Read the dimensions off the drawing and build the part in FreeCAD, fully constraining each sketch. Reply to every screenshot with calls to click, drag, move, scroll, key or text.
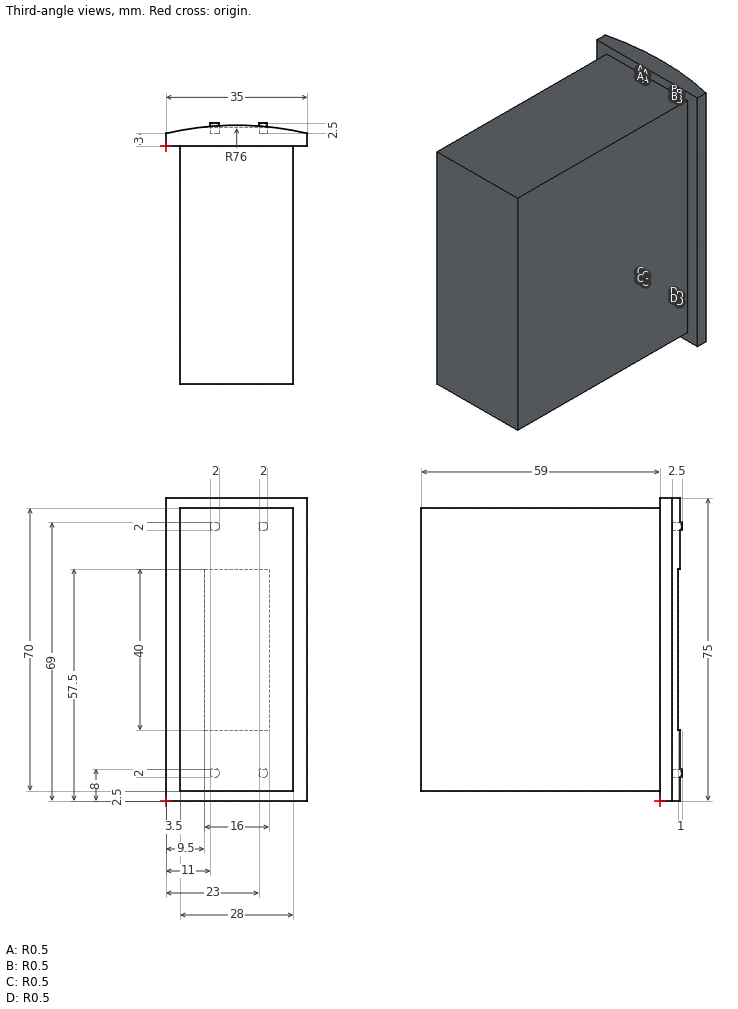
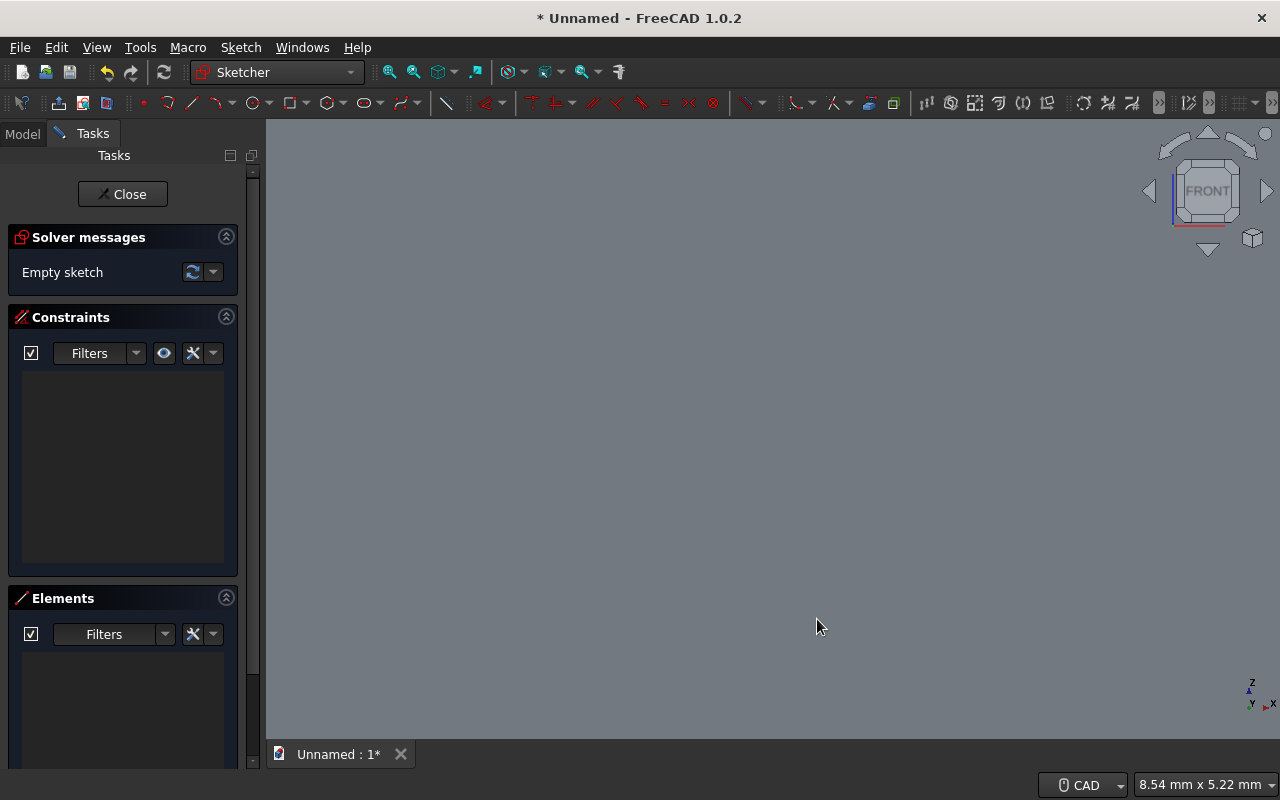
scroll(682, 380, up, 3)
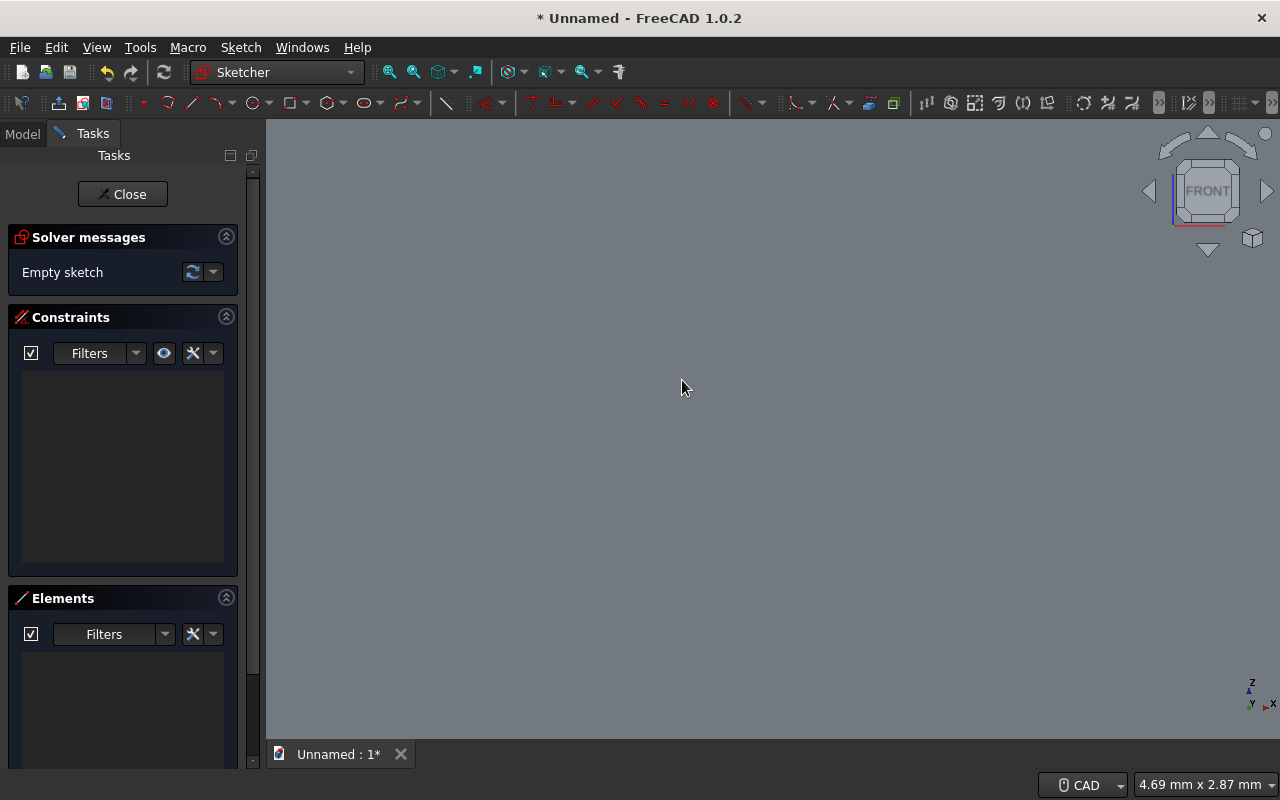
click(290, 104)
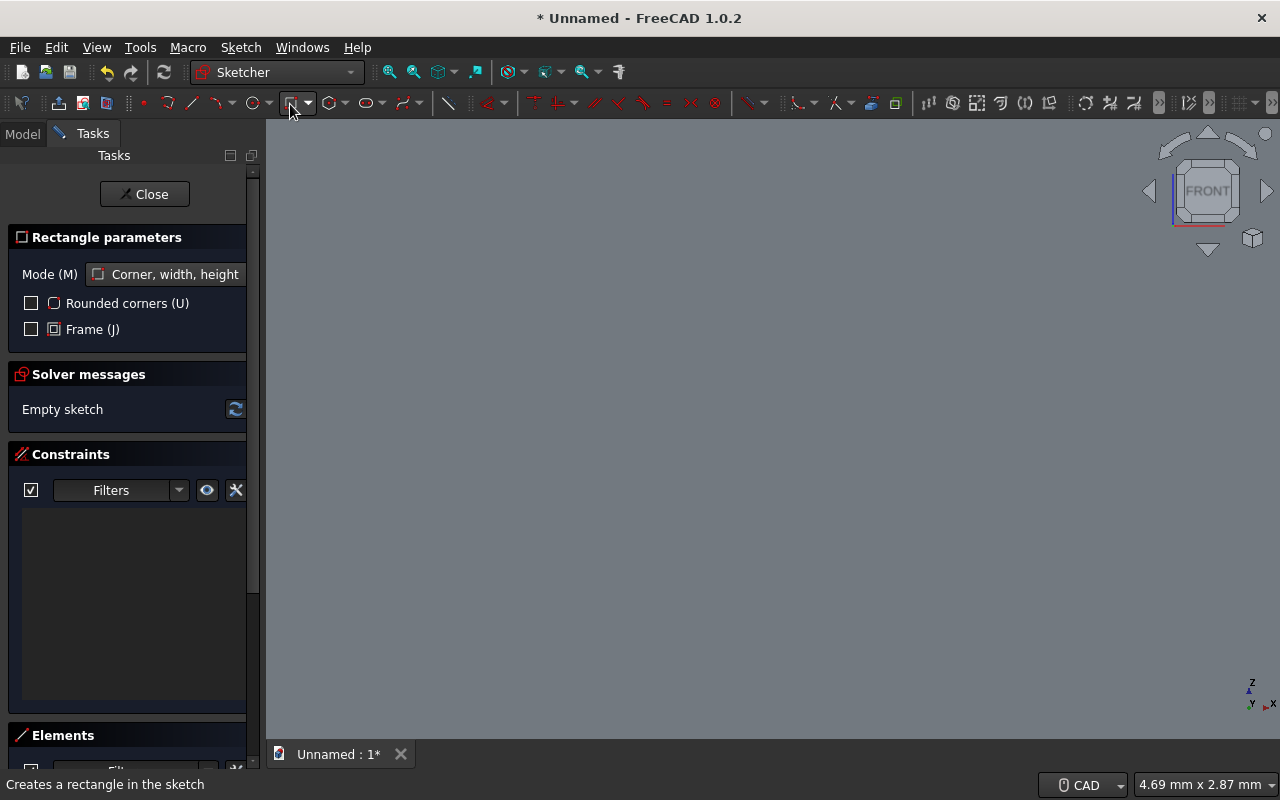
click(488, 213)
click(920, 645)
key(Escape)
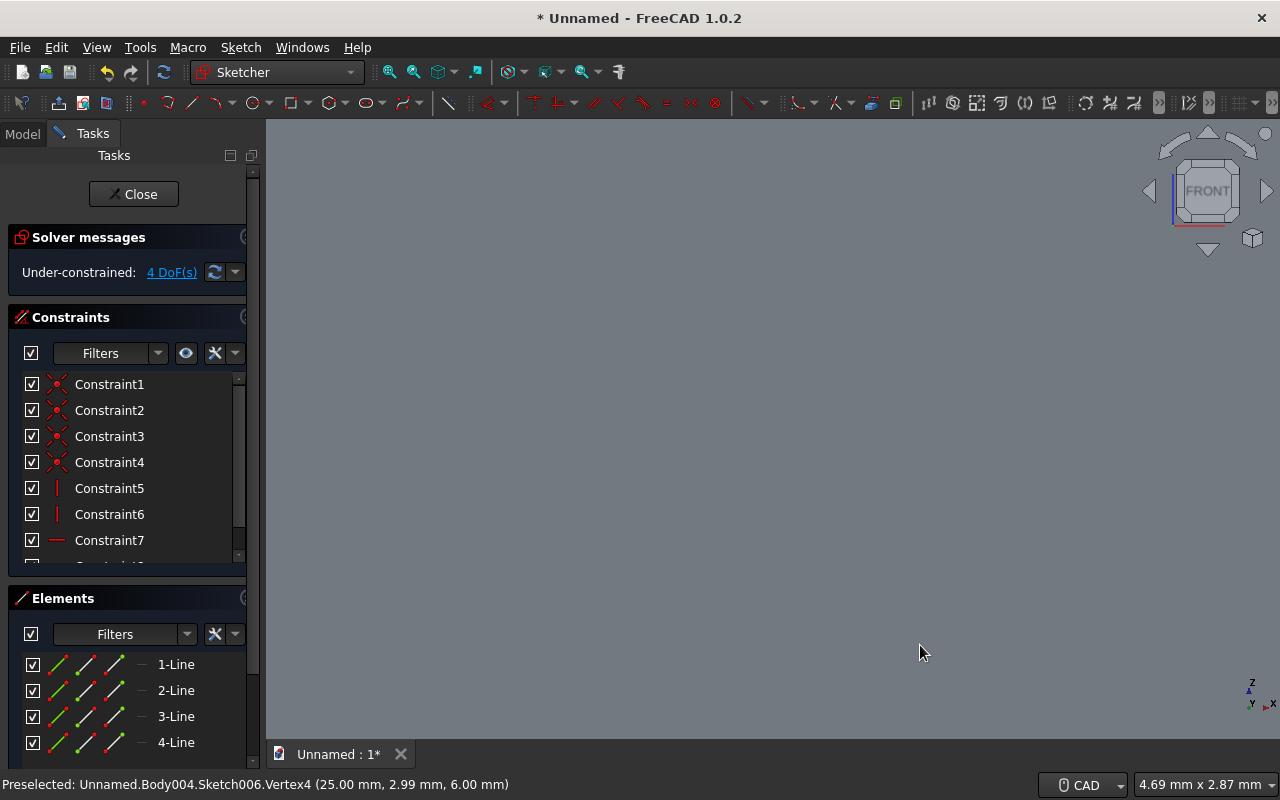
key(d)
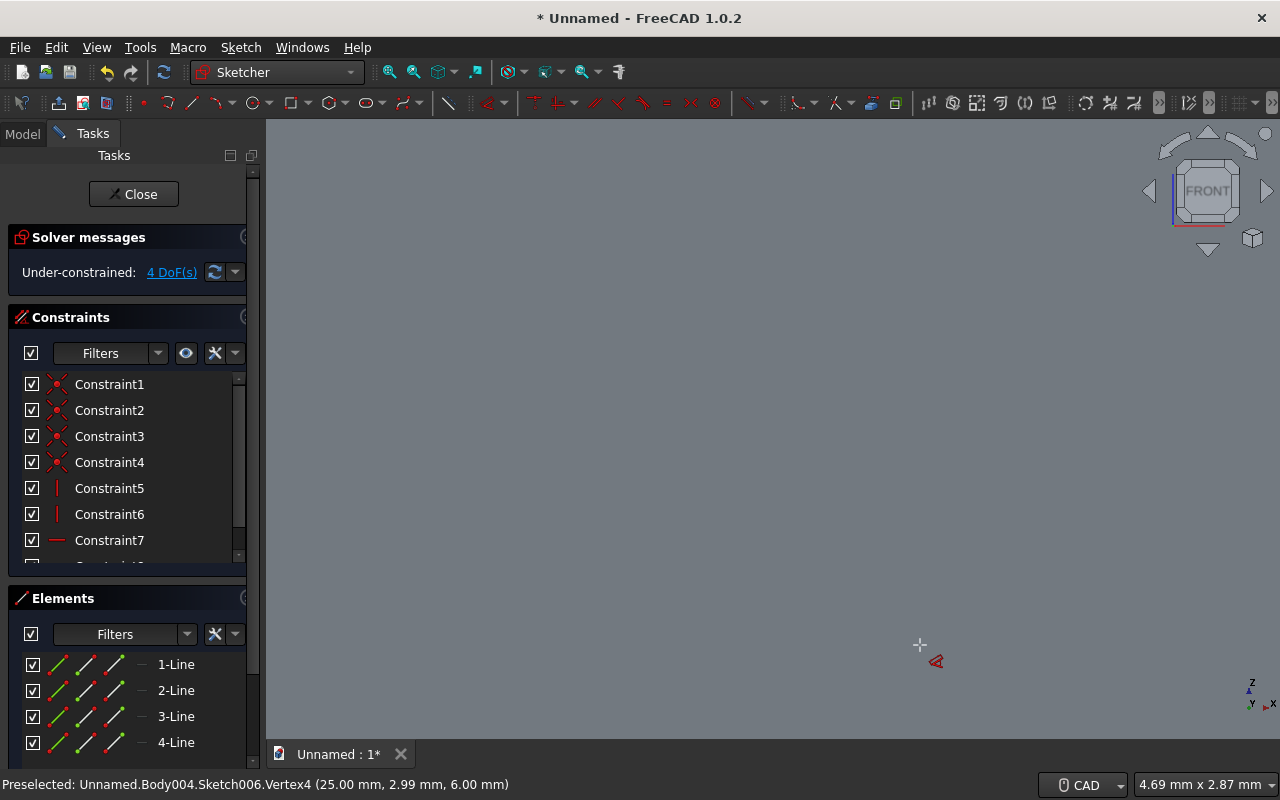
click(488, 344)
click(454, 430)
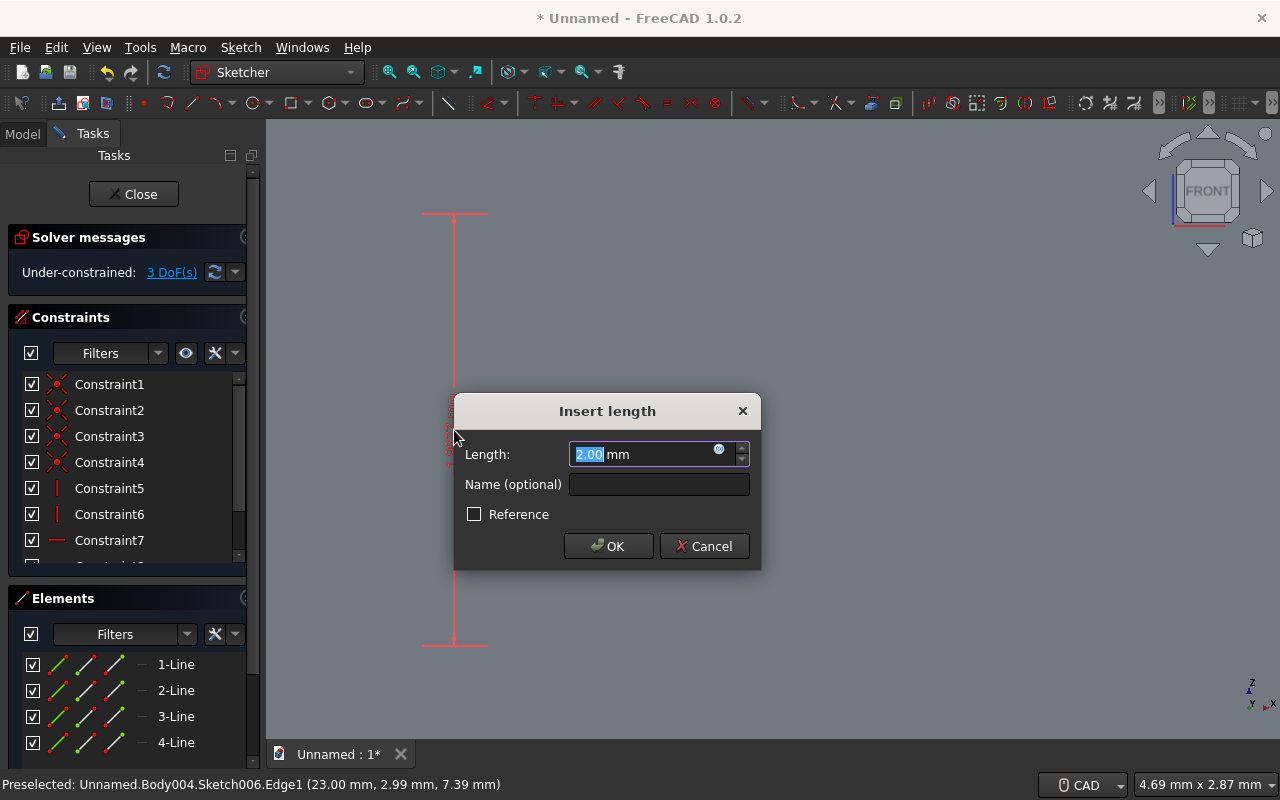
text(2)
key(Return)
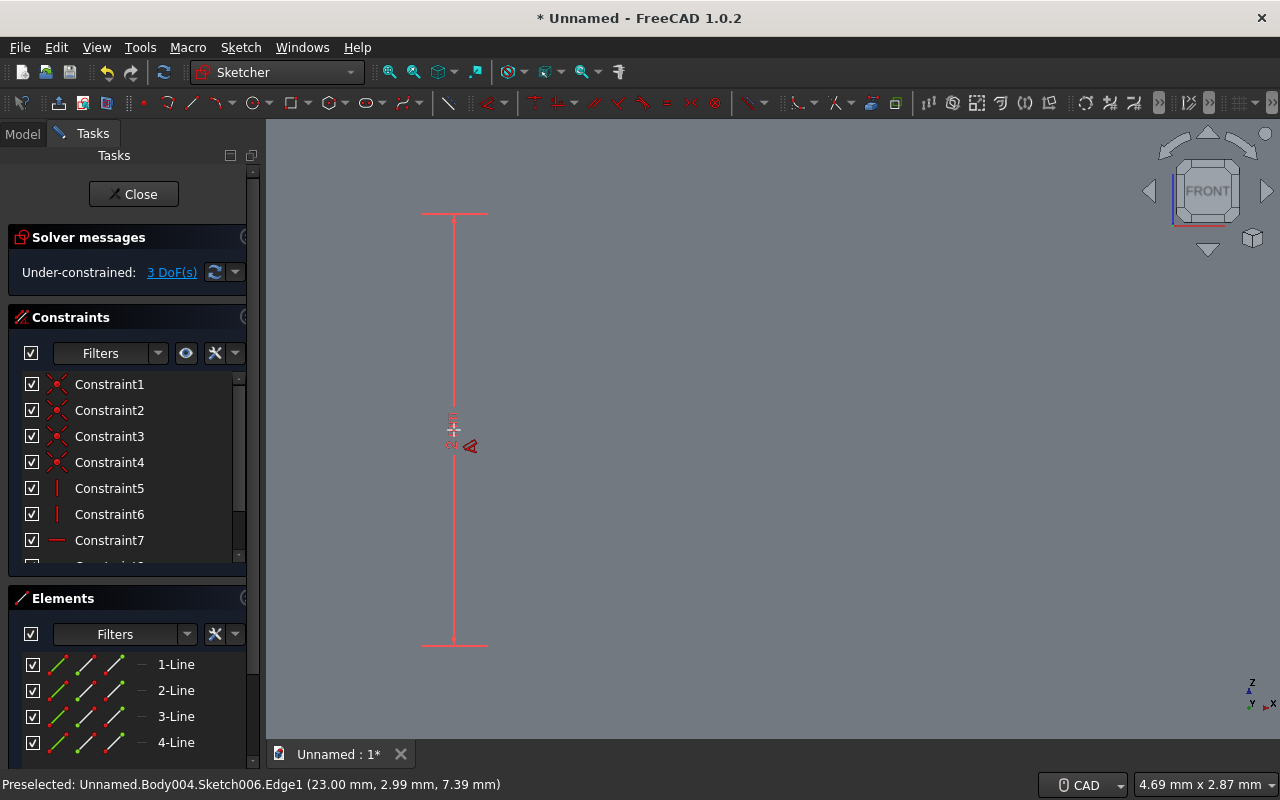
click(618, 646)
click(704, 680)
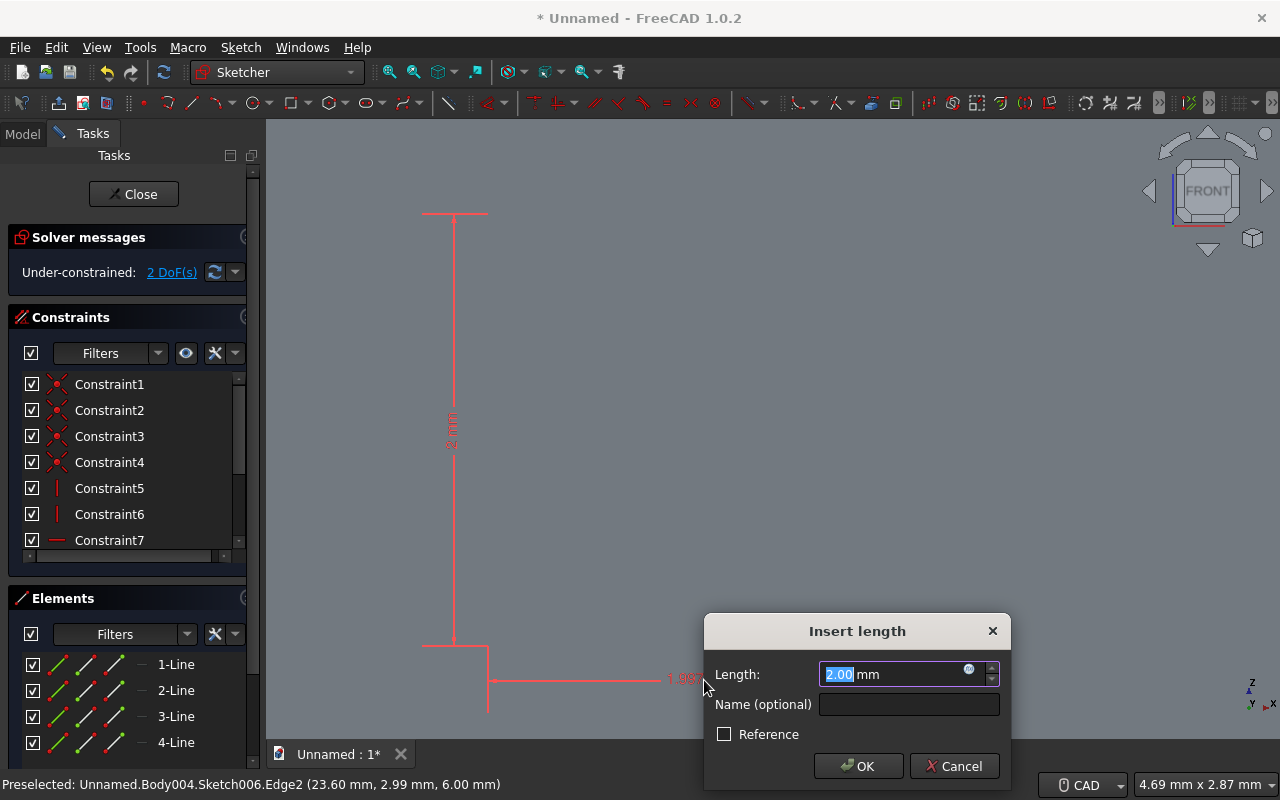
text(2)
key(Return)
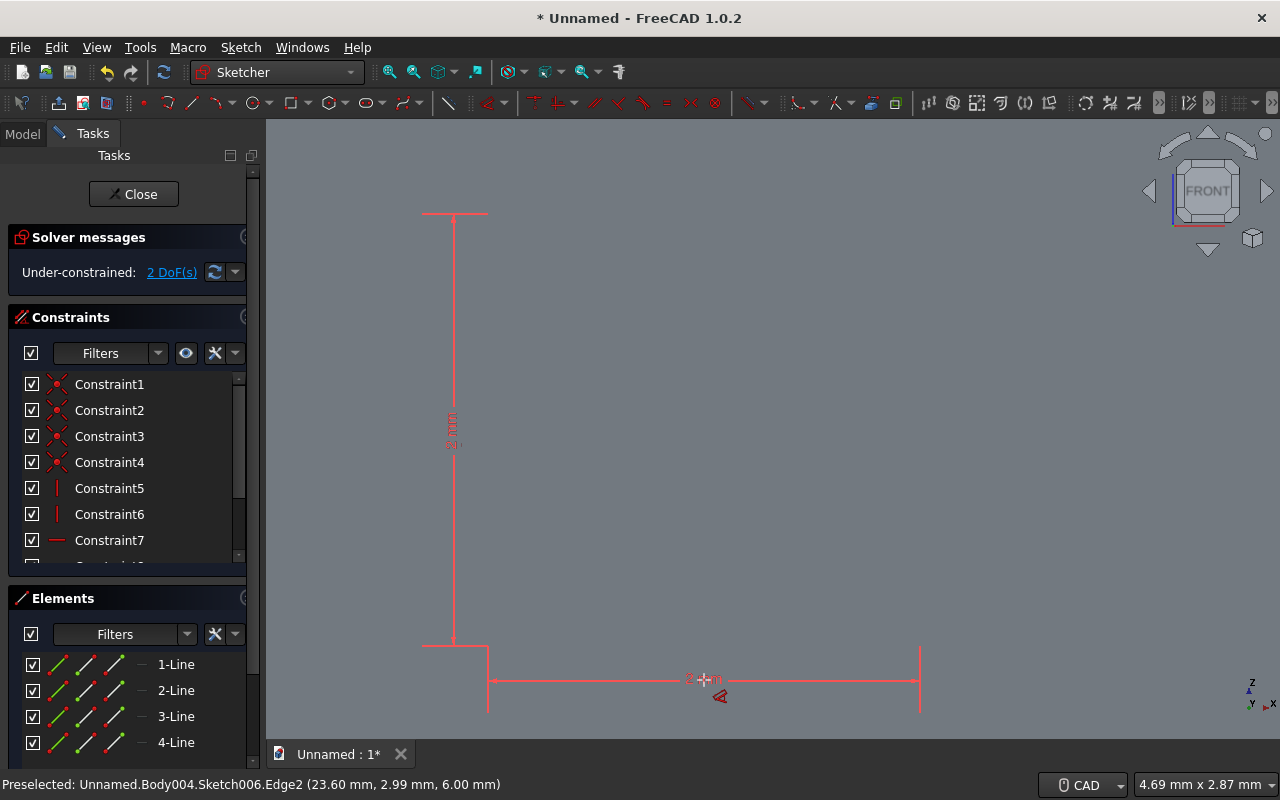
click(488, 214)
click(522, 462)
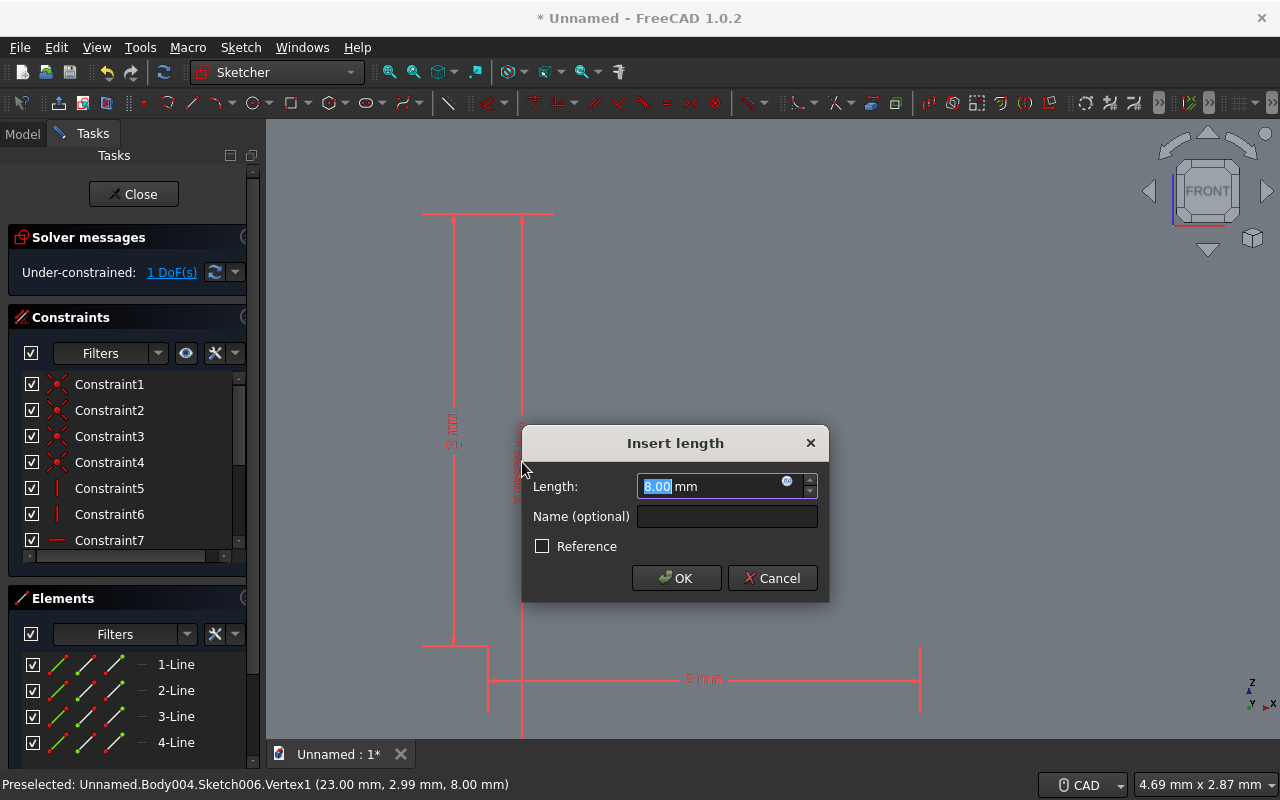
text(8)
key(Return)